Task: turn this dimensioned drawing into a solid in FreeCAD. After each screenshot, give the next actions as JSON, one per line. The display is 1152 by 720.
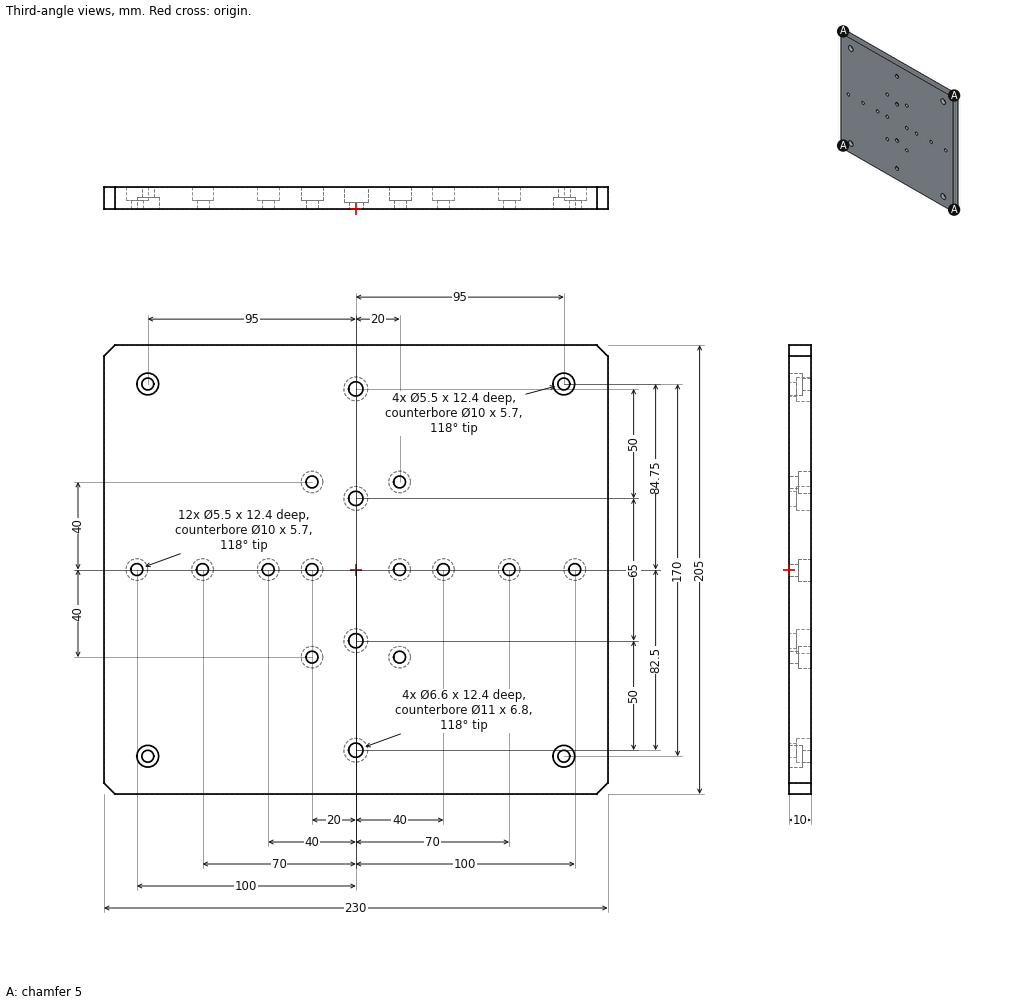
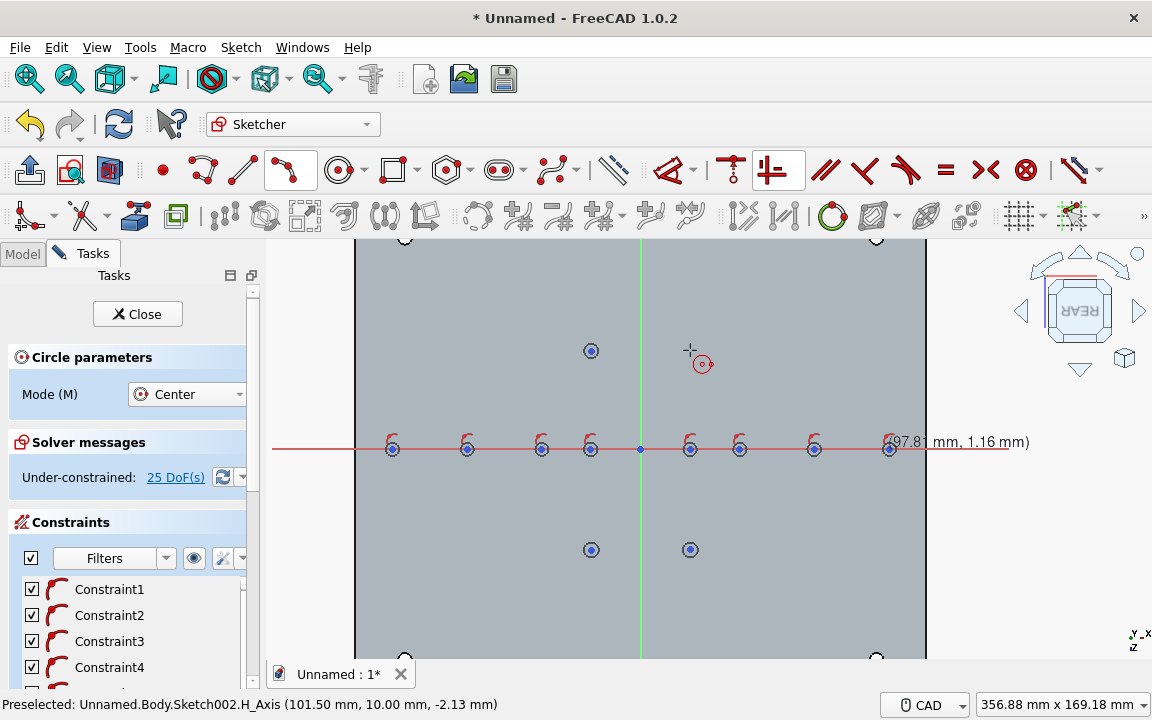
{"action": "left_click", "coordinate": [690, 350]}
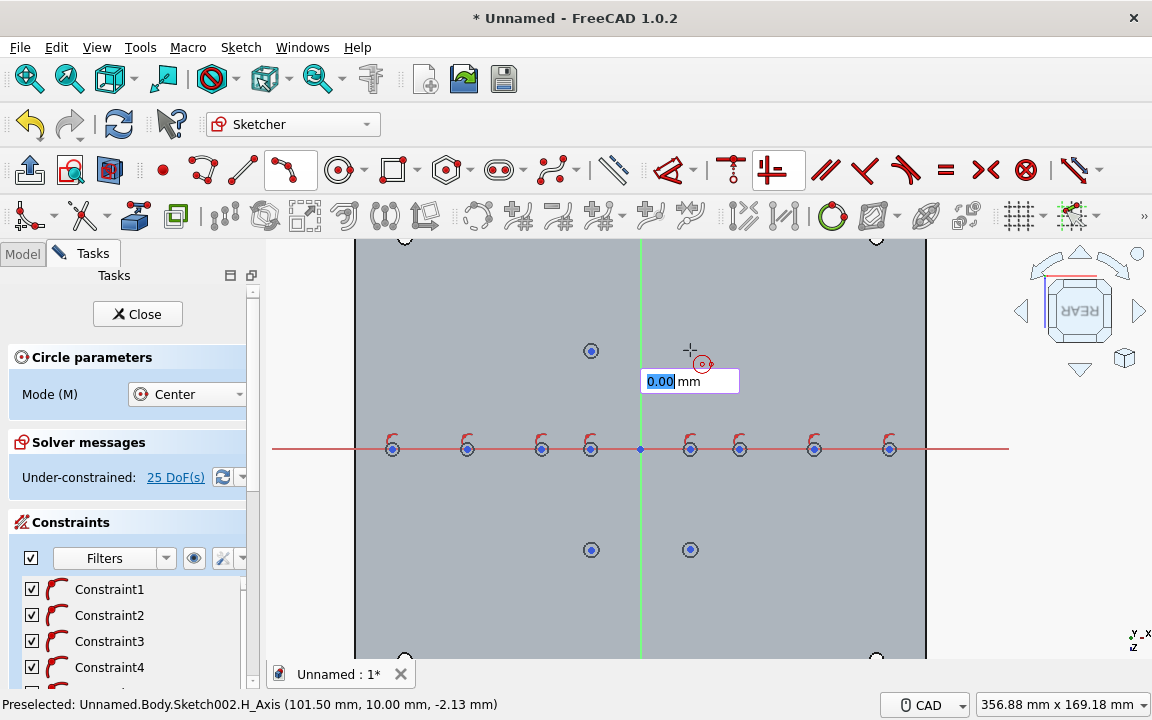
{"action": "scroll", "coordinate": [695, 345], "scroll_direction": "up", "scroll_amount": 5}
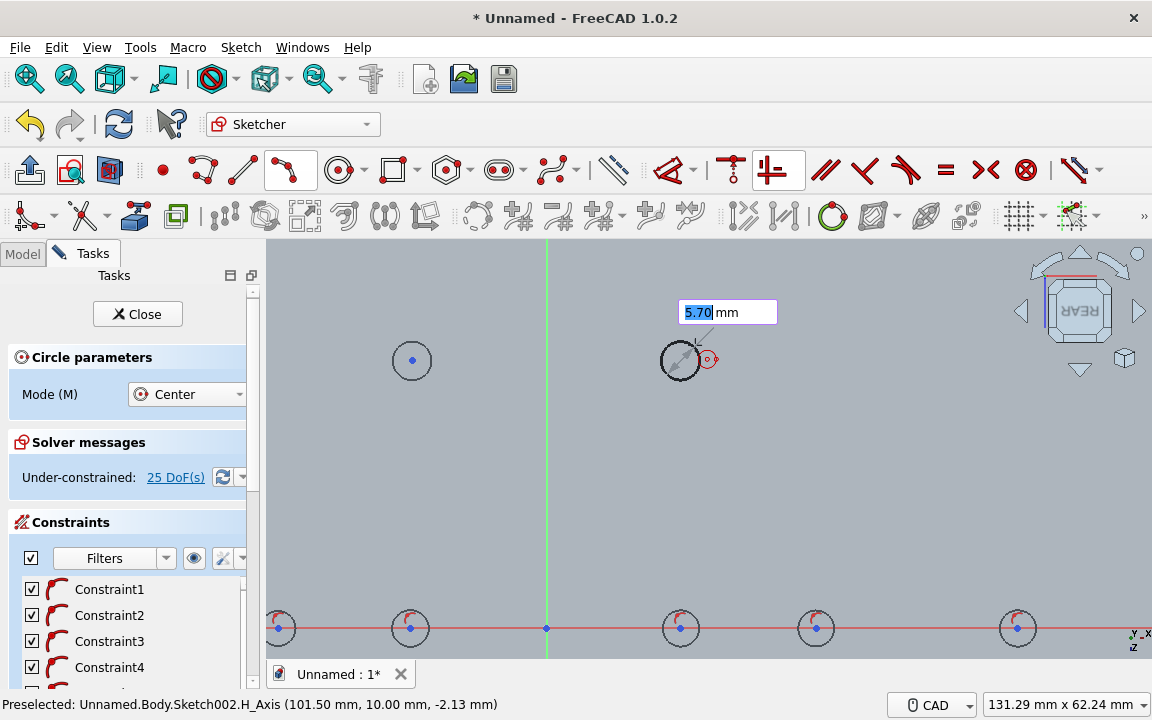
{"action": "left_click", "coordinate": [695, 345]}
{"action": "key", "text": "Escape"}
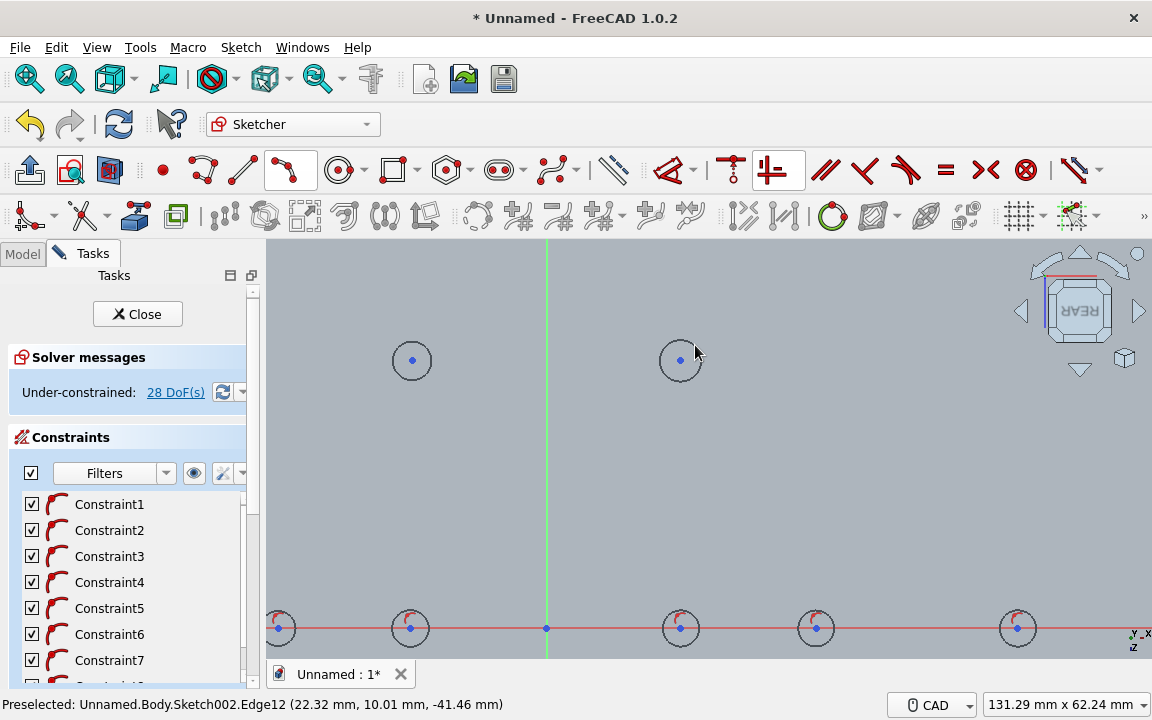
{"action": "scroll", "coordinate": [695, 345], "scroll_direction": "down", "scroll_amount": 5}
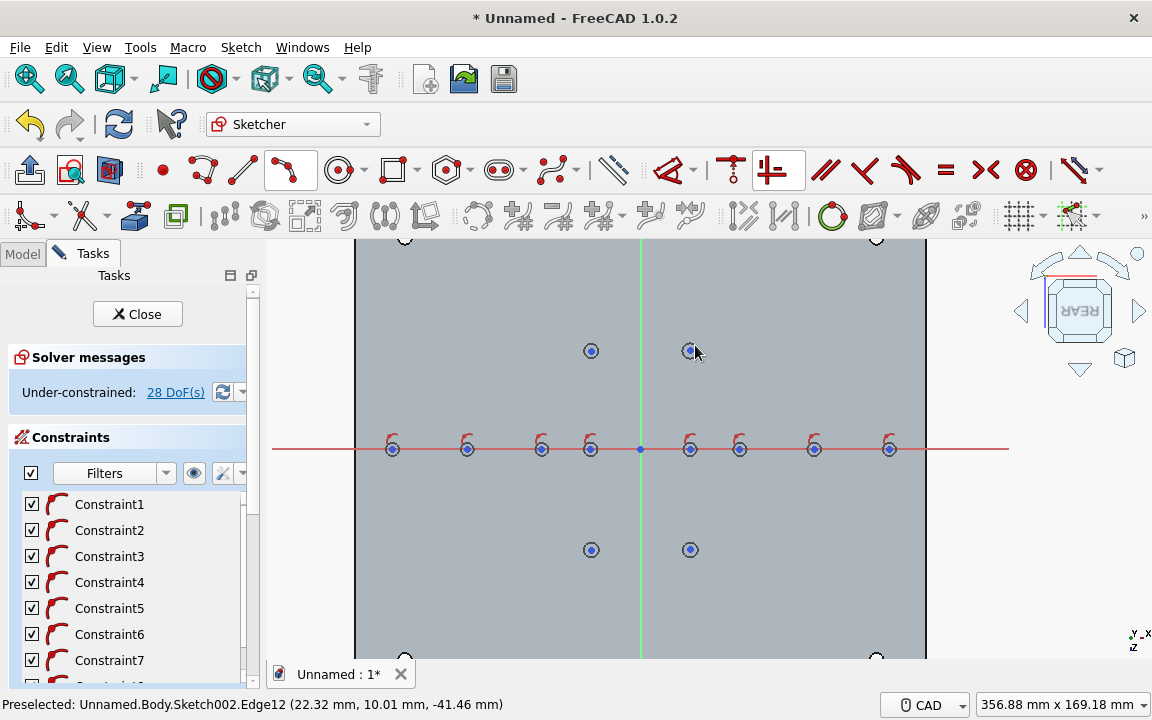
{"action": "scroll", "coordinate": [397, 445], "scroll_direction": "up", "scroll_amount": 6}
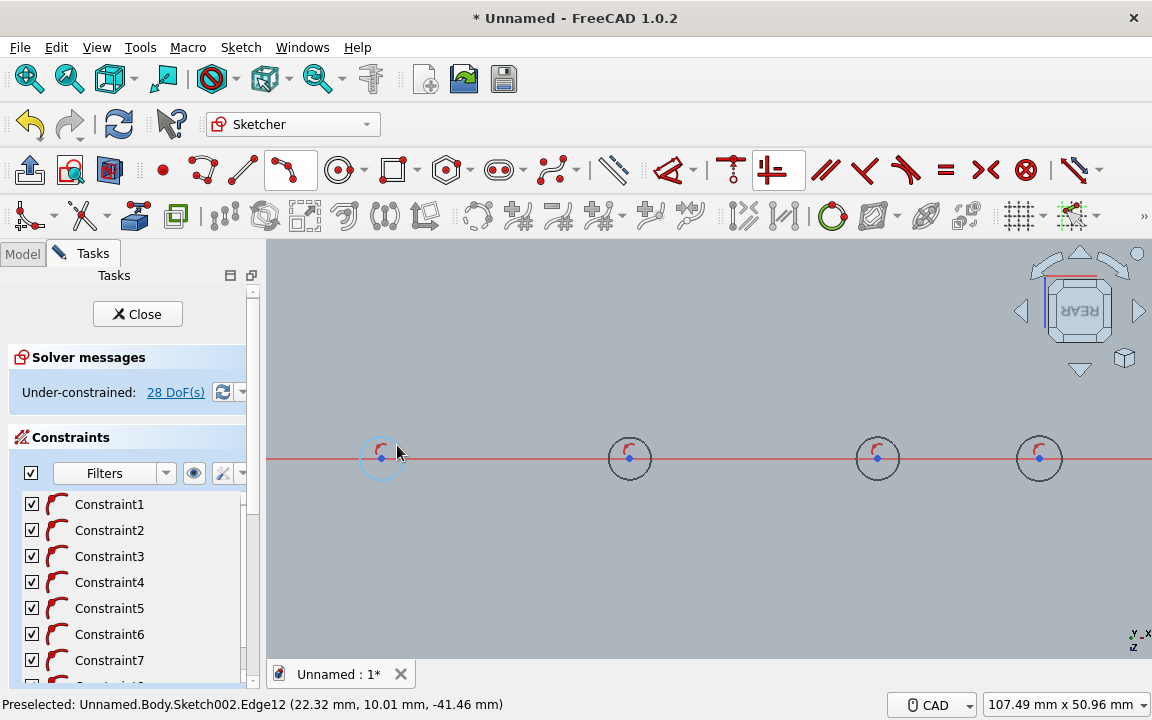
{"action": "left_click", "coordinate": [397, 443]}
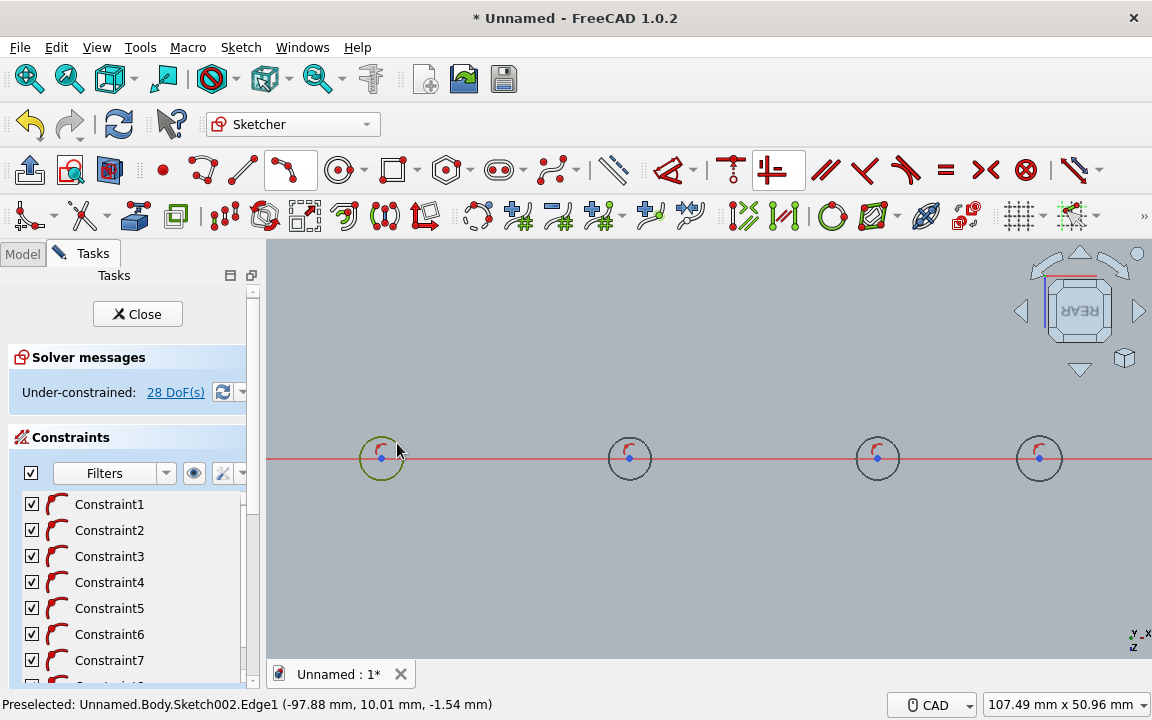
{"action": "left_click", "coordinate": [645, 444]}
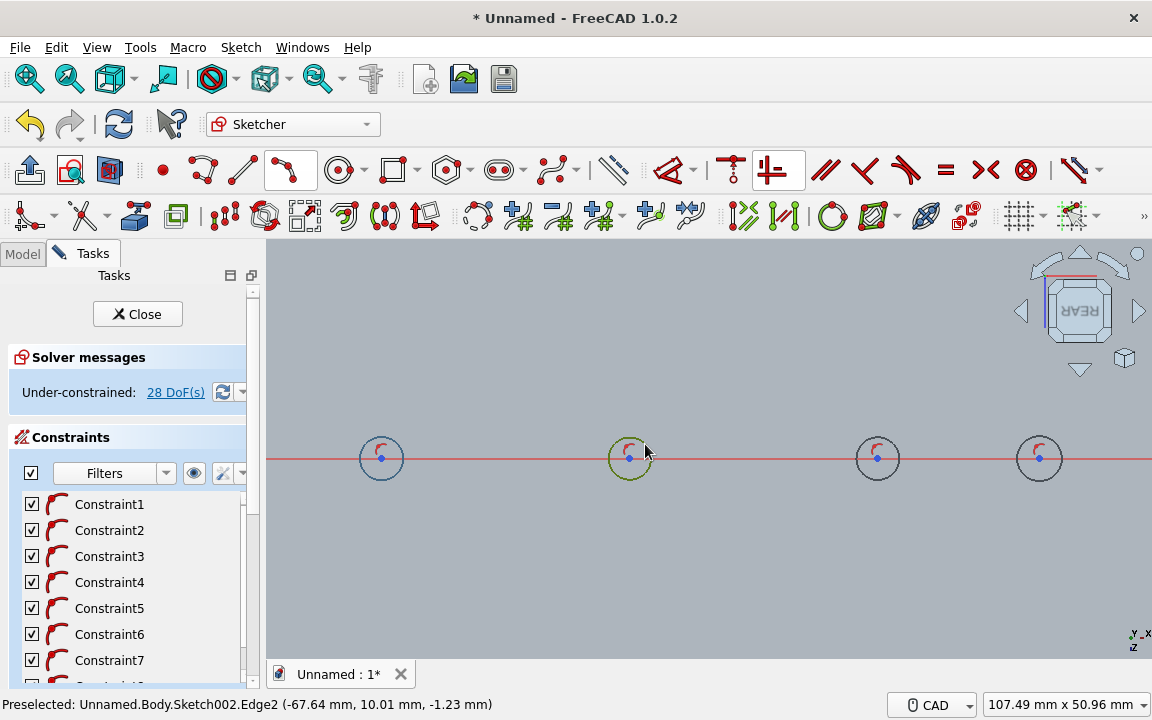
{"action": "left_click", "coordinate": [893, 443]}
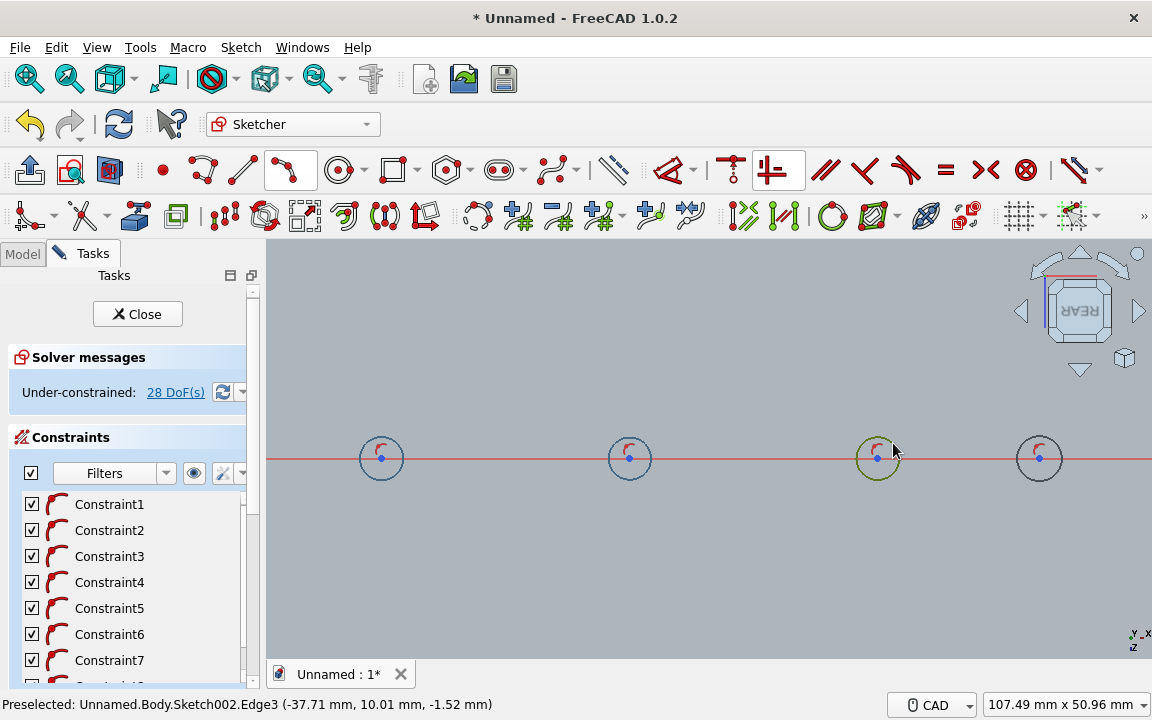
{"action": "scroll", "coordinate": [397, 445], "scroll_direction": "down", "scroll_amount": 6}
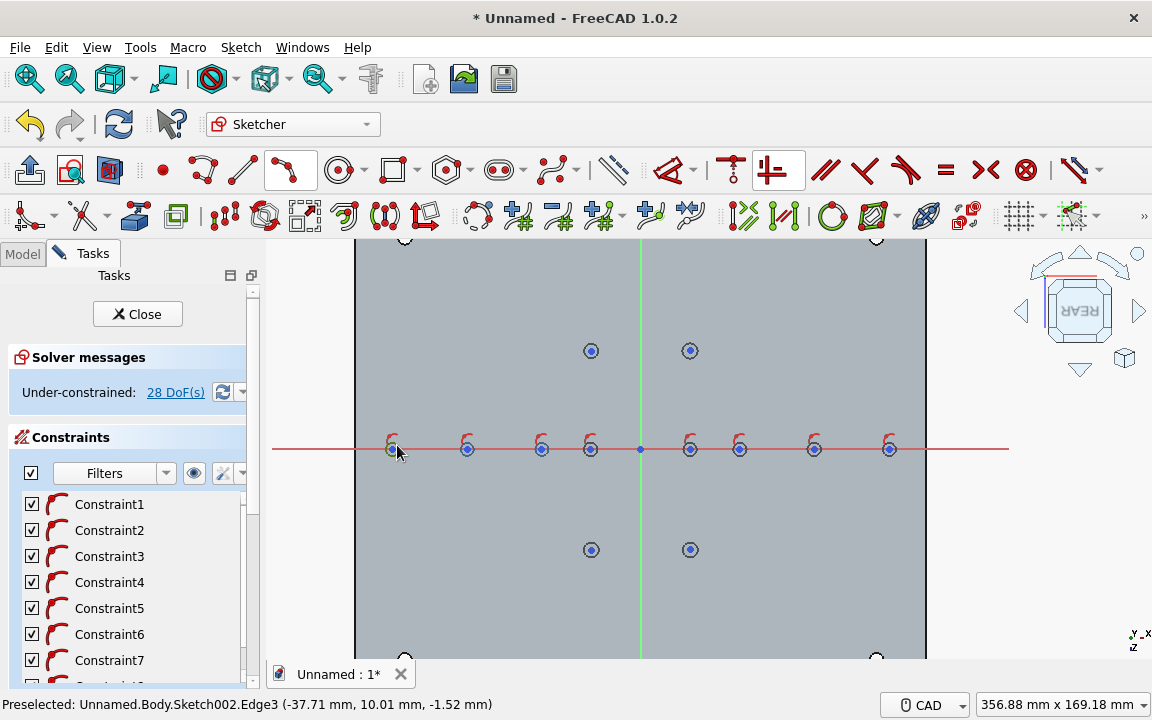
{"action": "scroll", "coordinate": [595, 445], "scroll_direction": "up", "scroll_amount": 6}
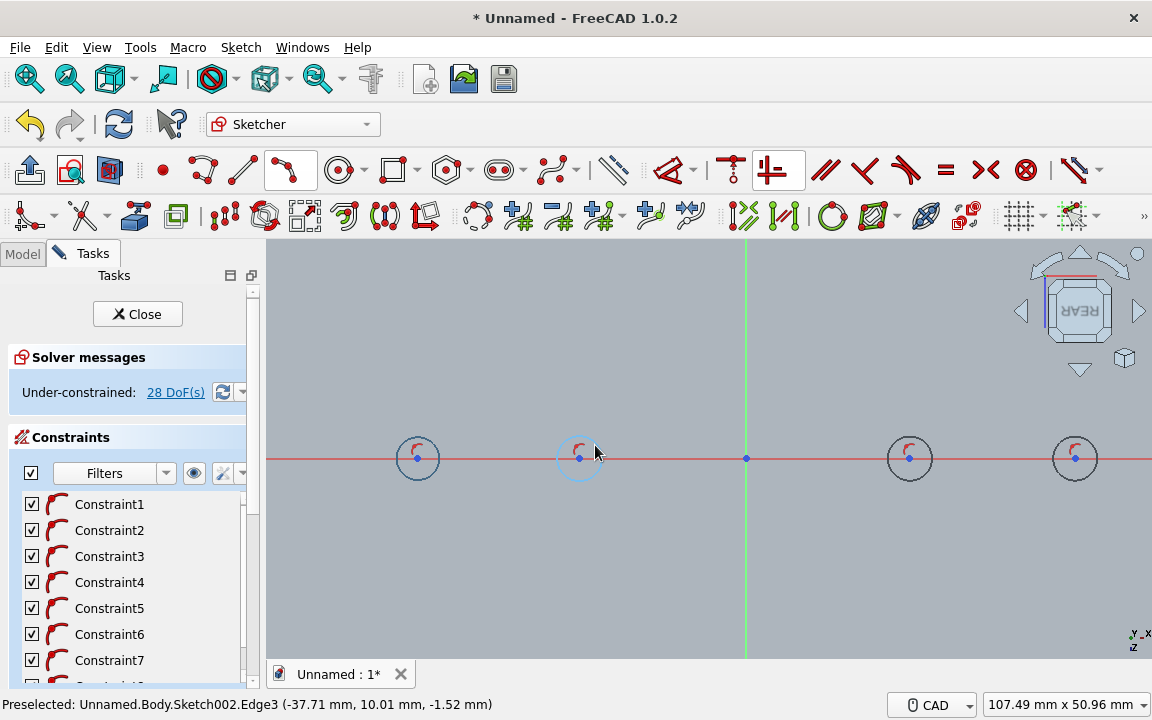
{"action": "left_click", "coordinate": [595, 443]}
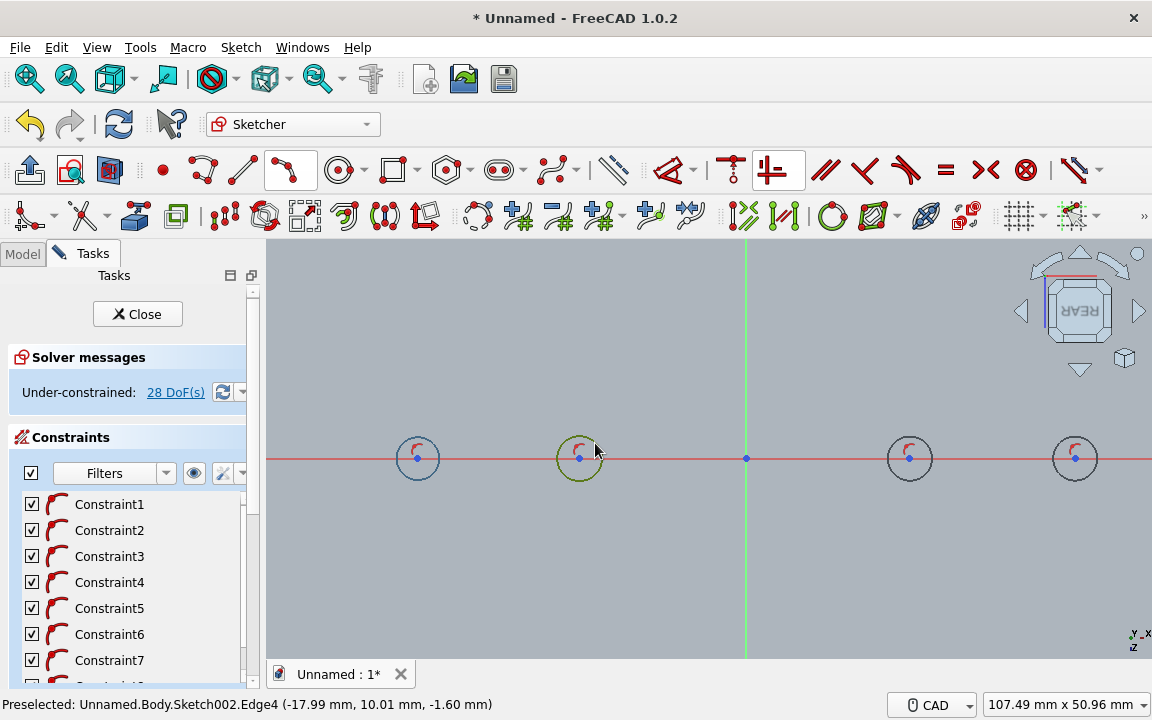
{"action": "scroll", "coordinate": [595, 445], "scroll_direction": "down", "scroll_amount": 6}